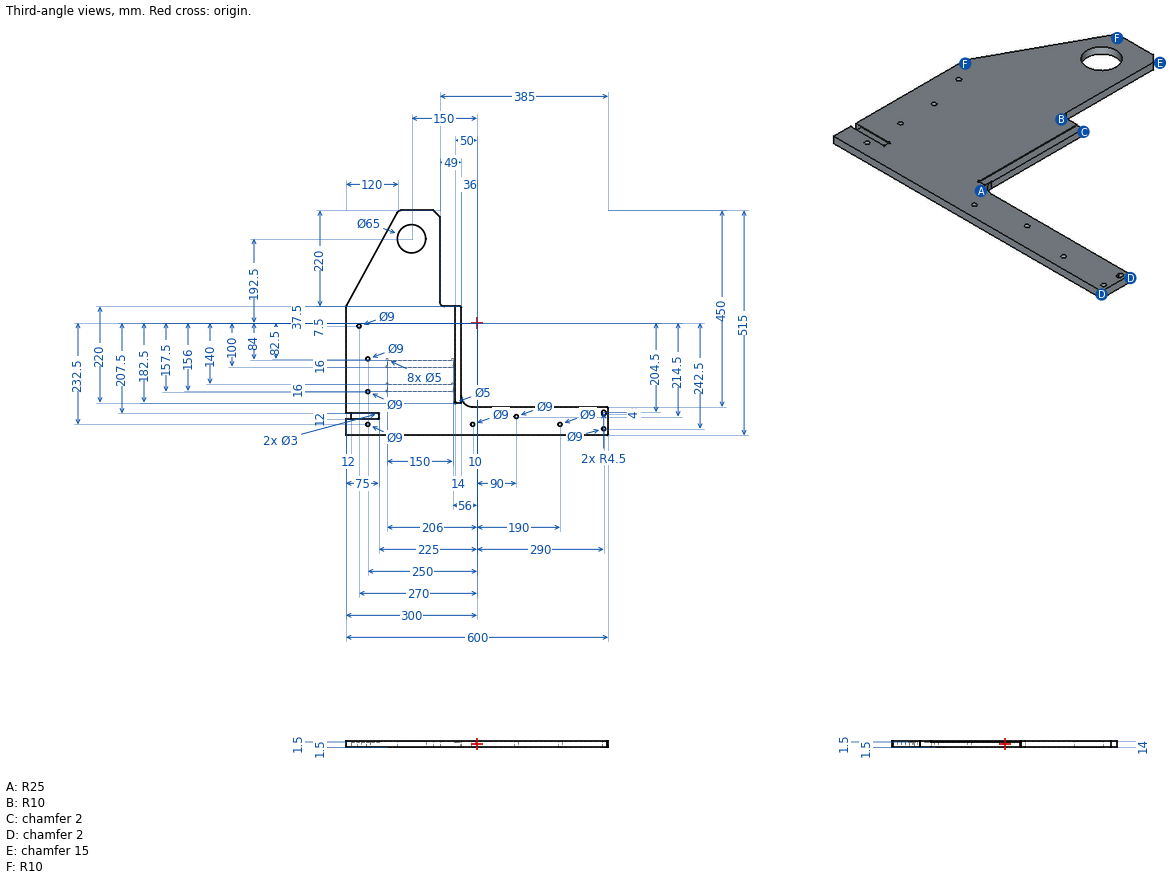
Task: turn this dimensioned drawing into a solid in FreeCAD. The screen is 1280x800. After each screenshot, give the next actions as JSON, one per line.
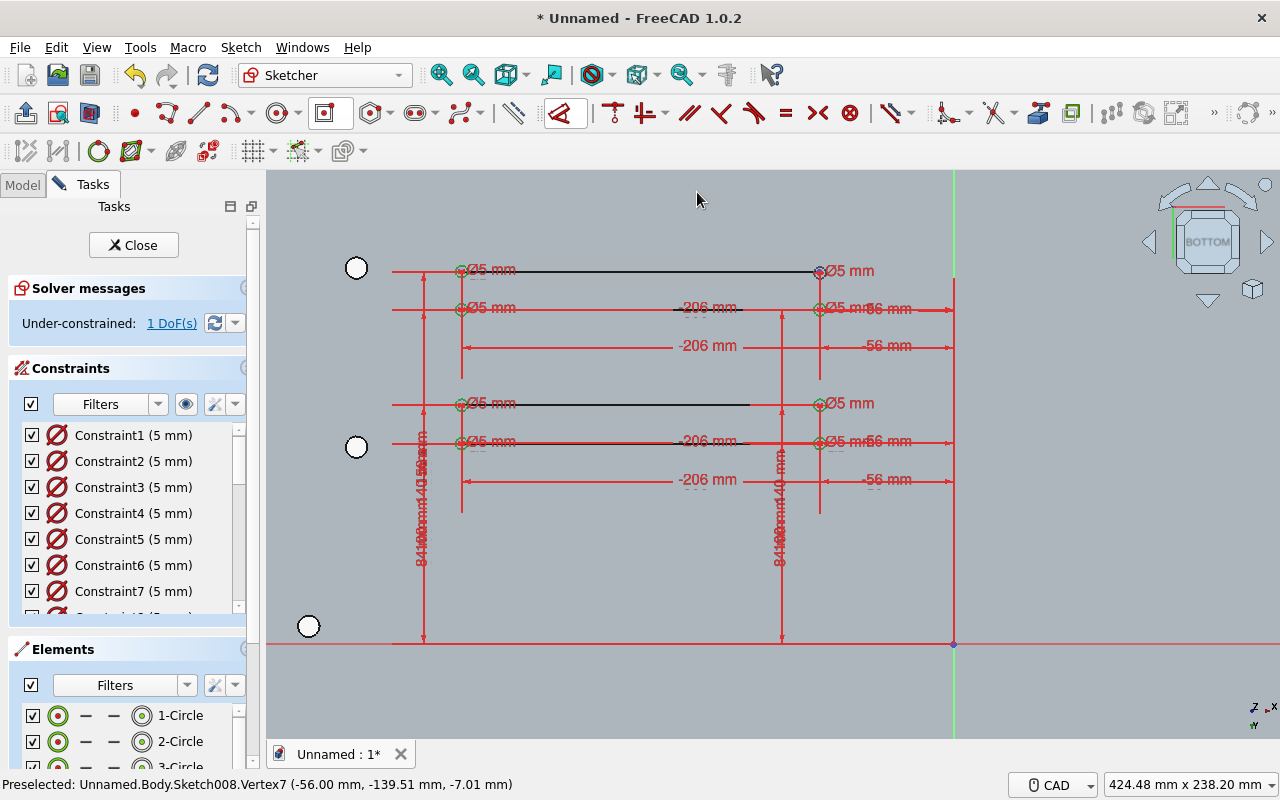
{"action": "left_click", "coordinate": [820, 273]}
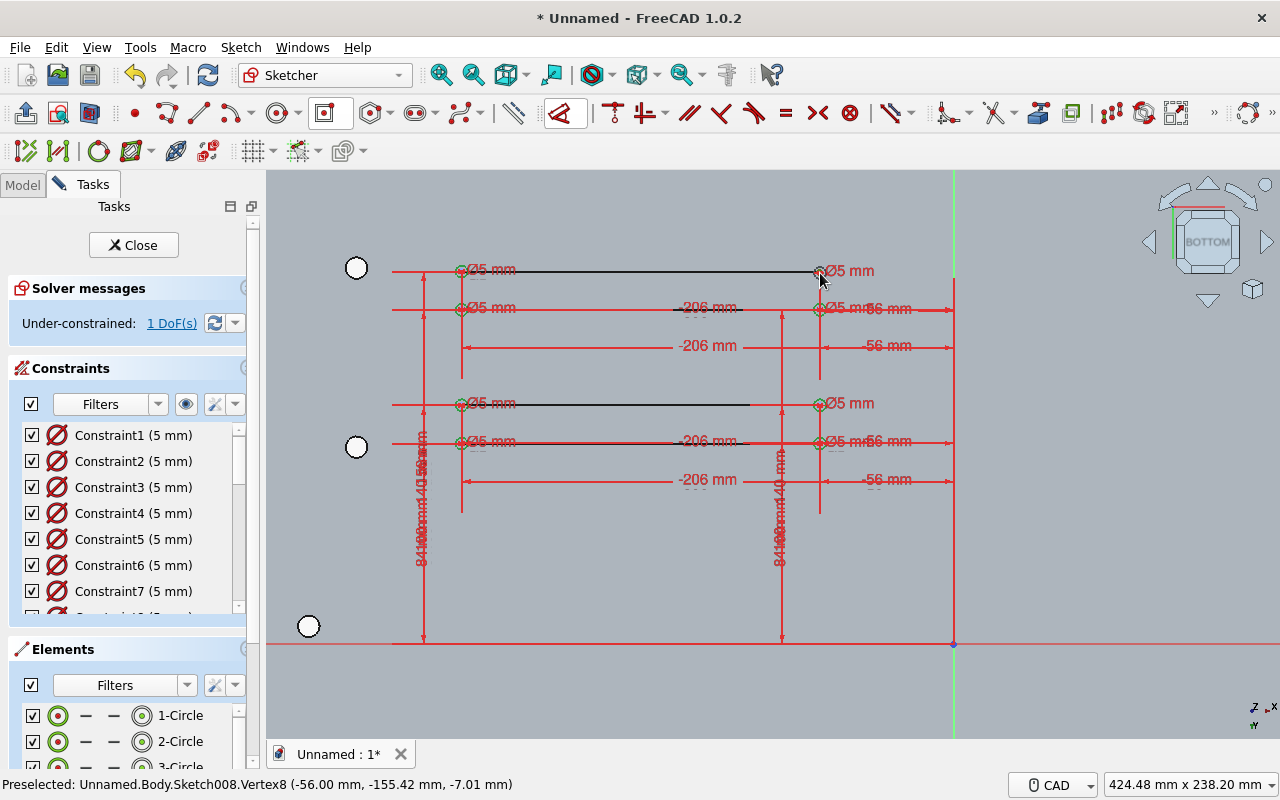
{"action": "key", "text": "i"}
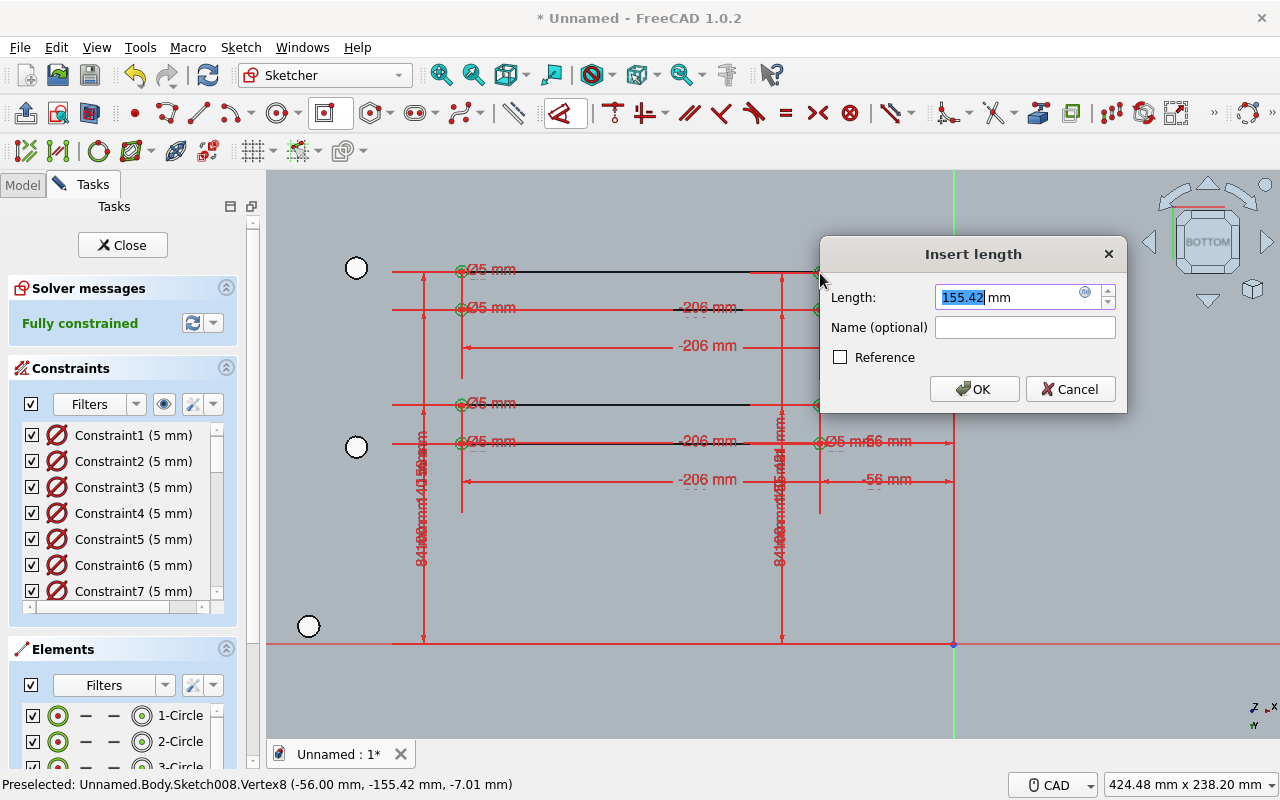
{"action": "type", "text": "156"}
{"action": "key", "text": "Return"}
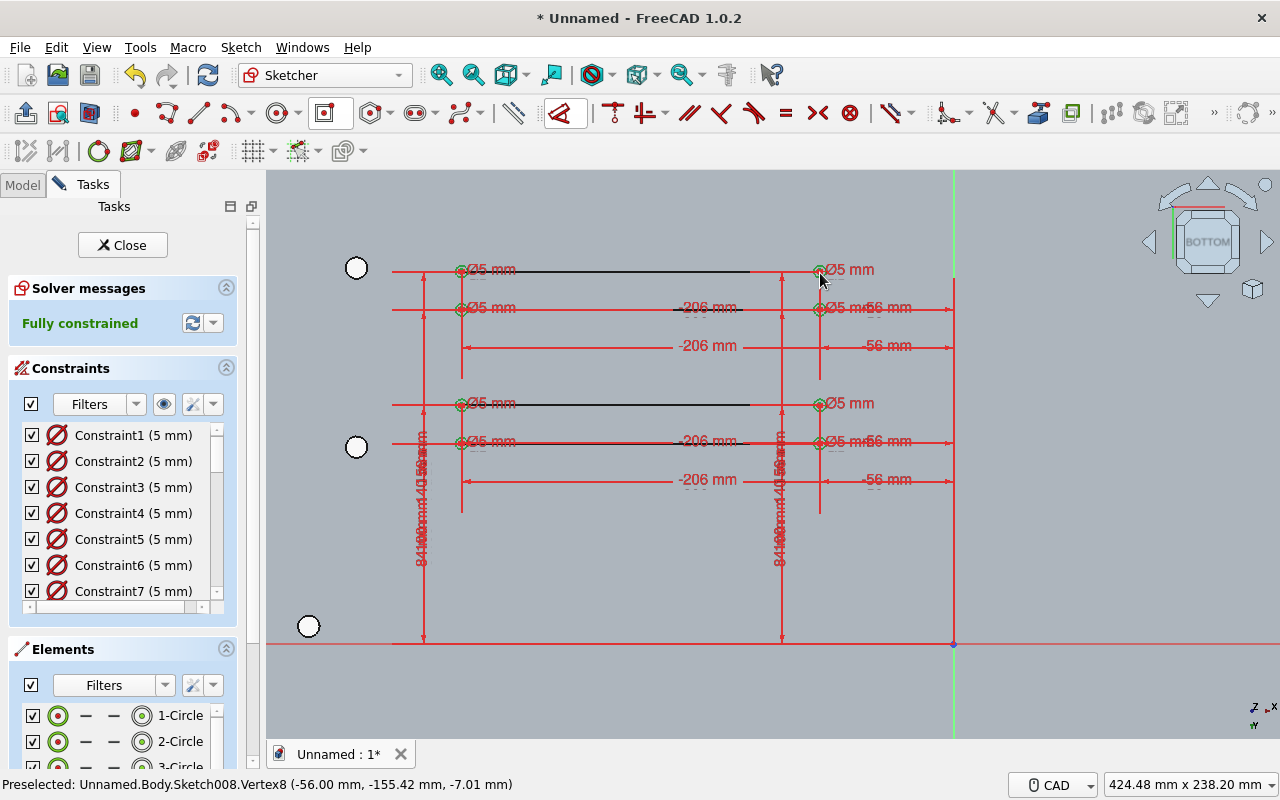
{"action": "left_click", "coordinate": [123, 245]}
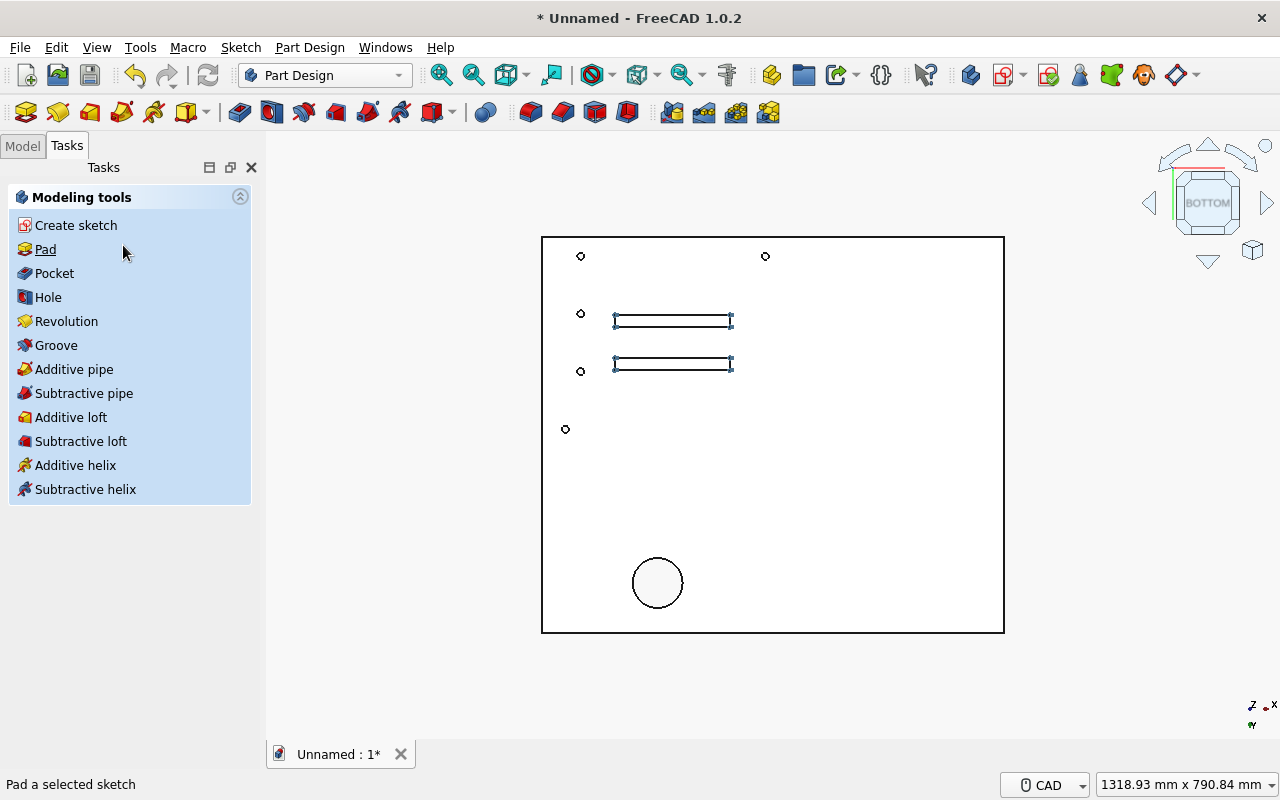
{"action": "left_click", "coordinate": [240, 112]}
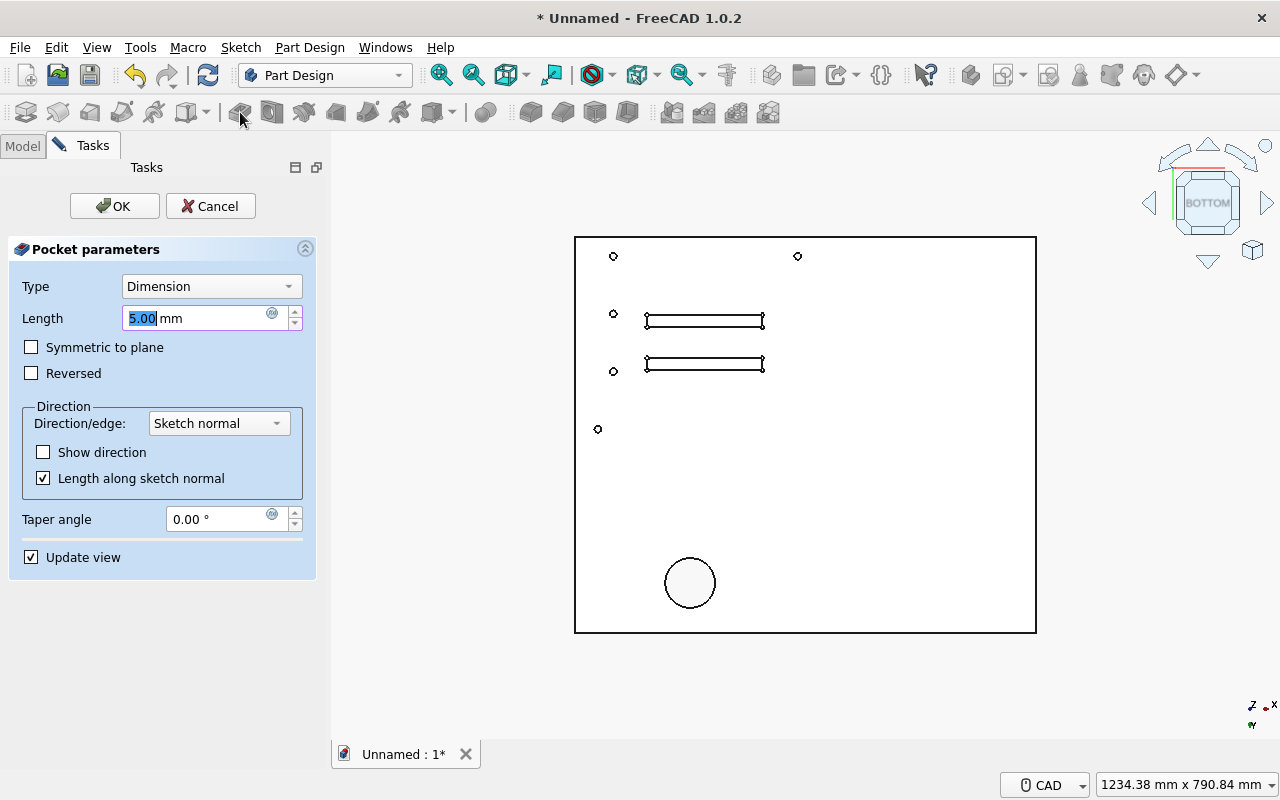
{"action": "type", "text": "1.5"}
{"action": "key", "text": "Tab"}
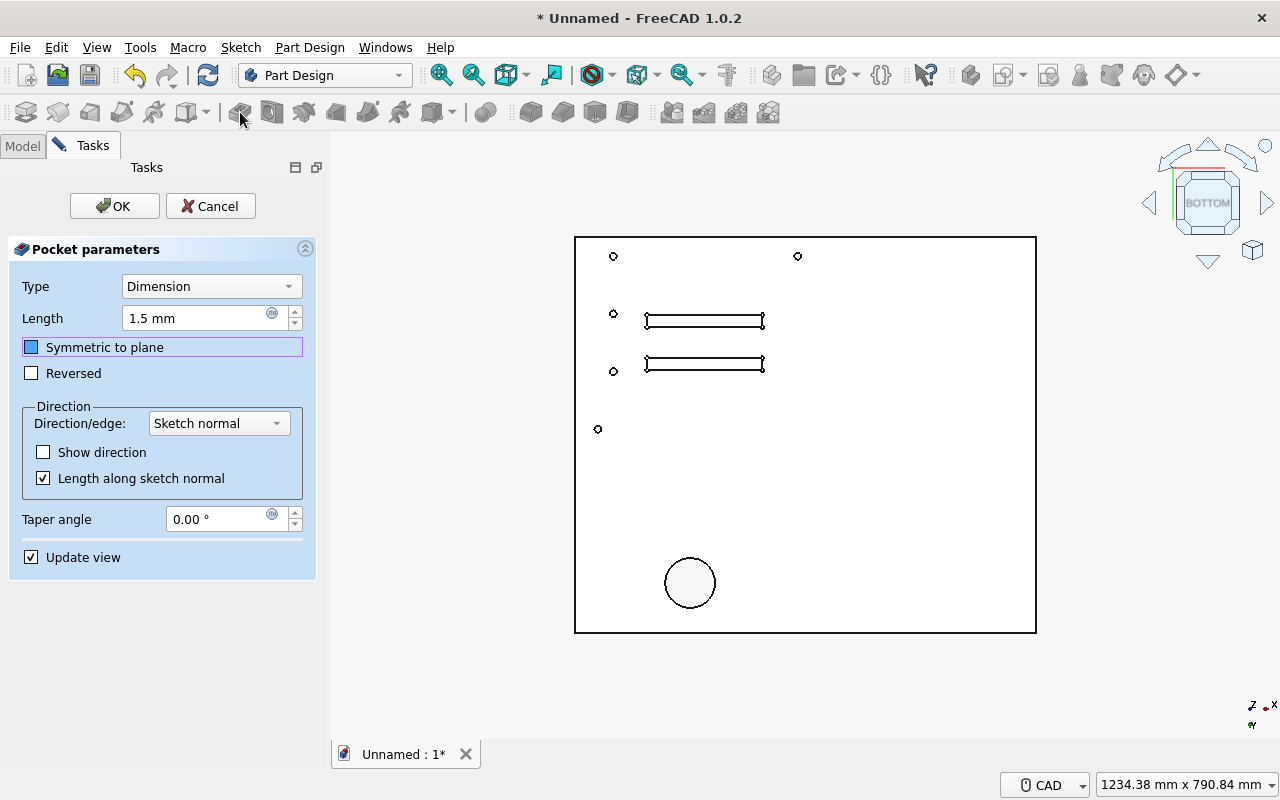
{"action": "left_click", "coordinate": [115, 206]}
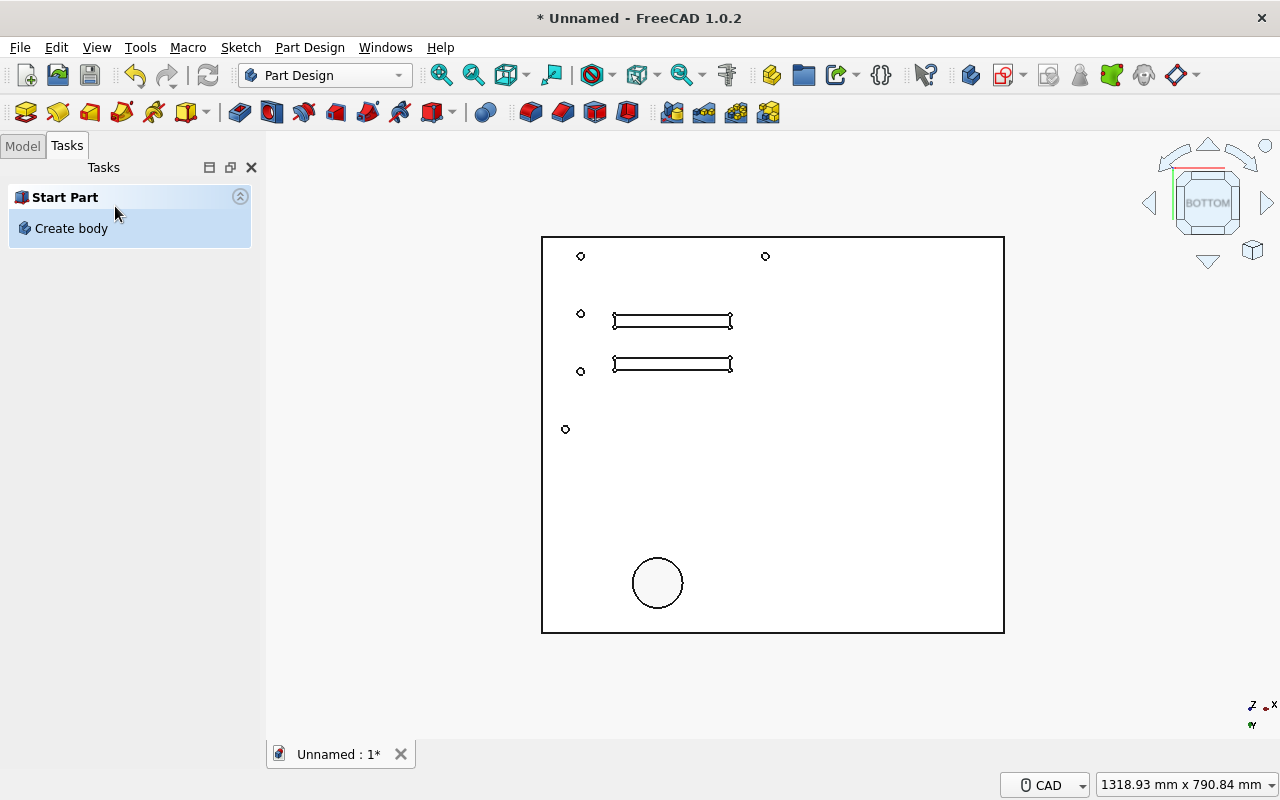
{"action": "key", "text": "0"}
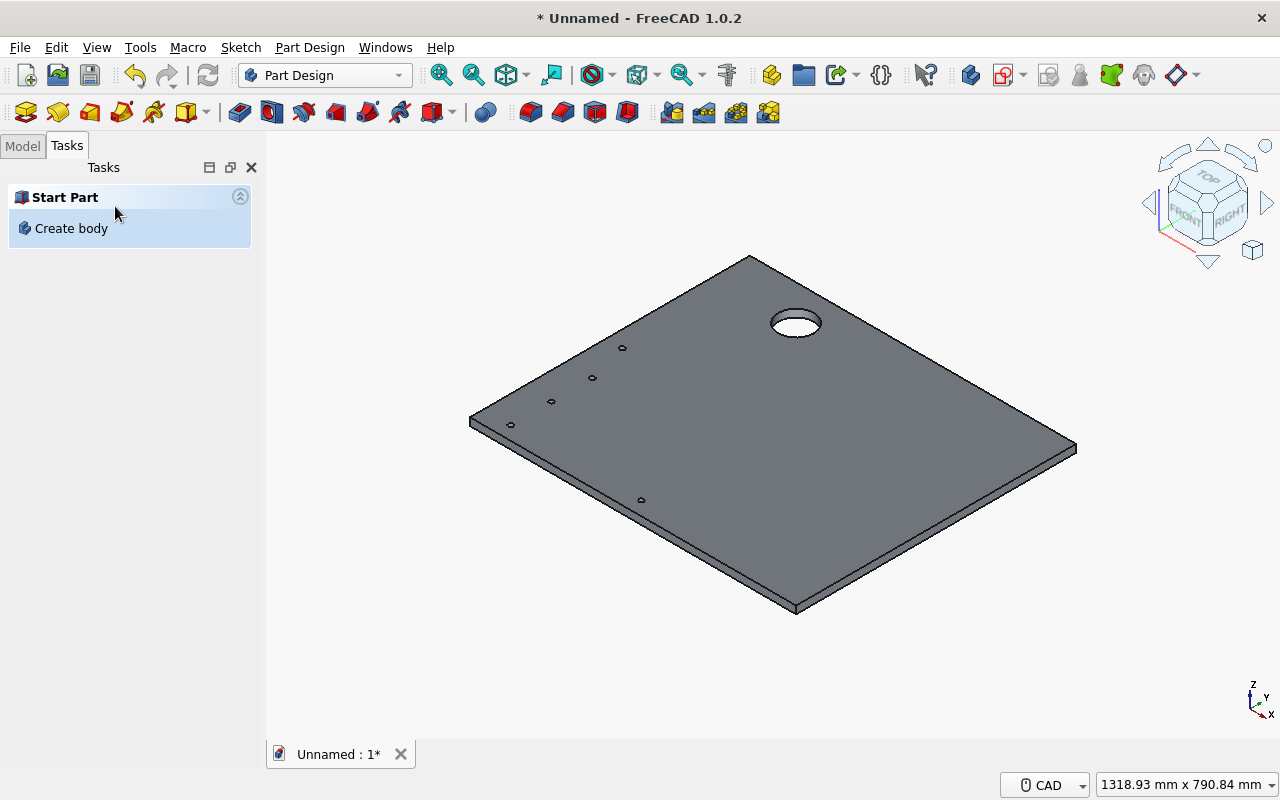
{"action": "left_click", "coordinate": [820, 457]}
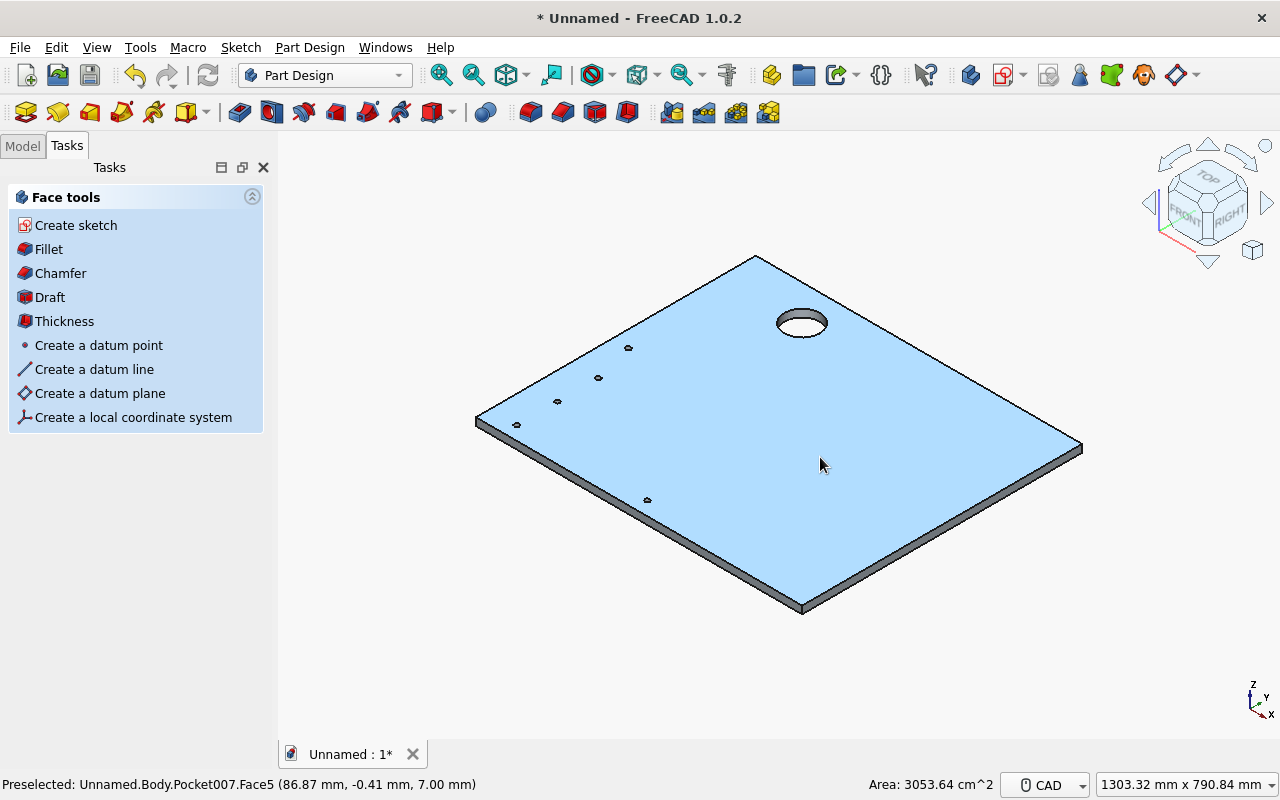
{"action": "left_click", "coordinate": [1004, 76]}